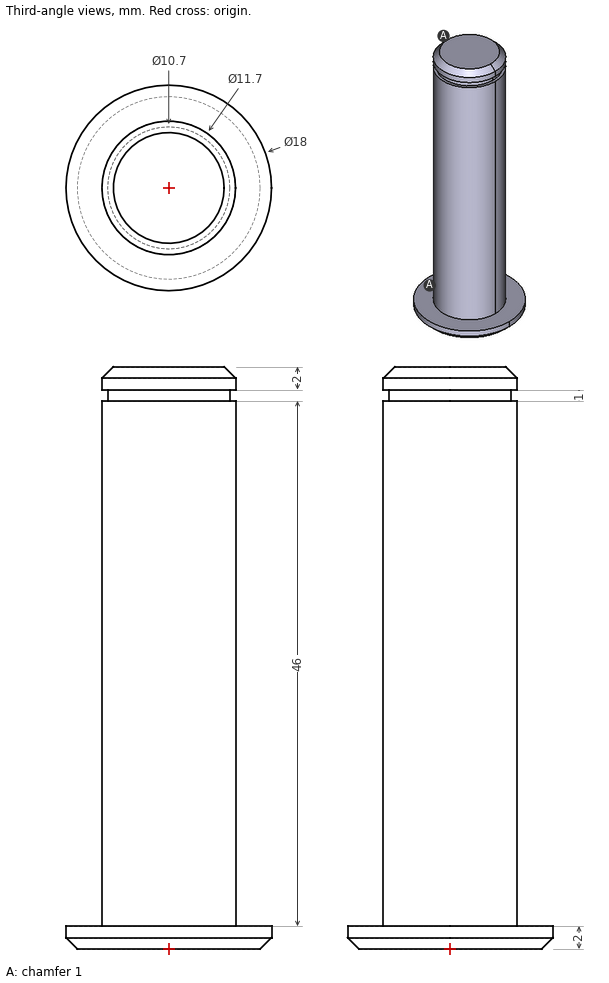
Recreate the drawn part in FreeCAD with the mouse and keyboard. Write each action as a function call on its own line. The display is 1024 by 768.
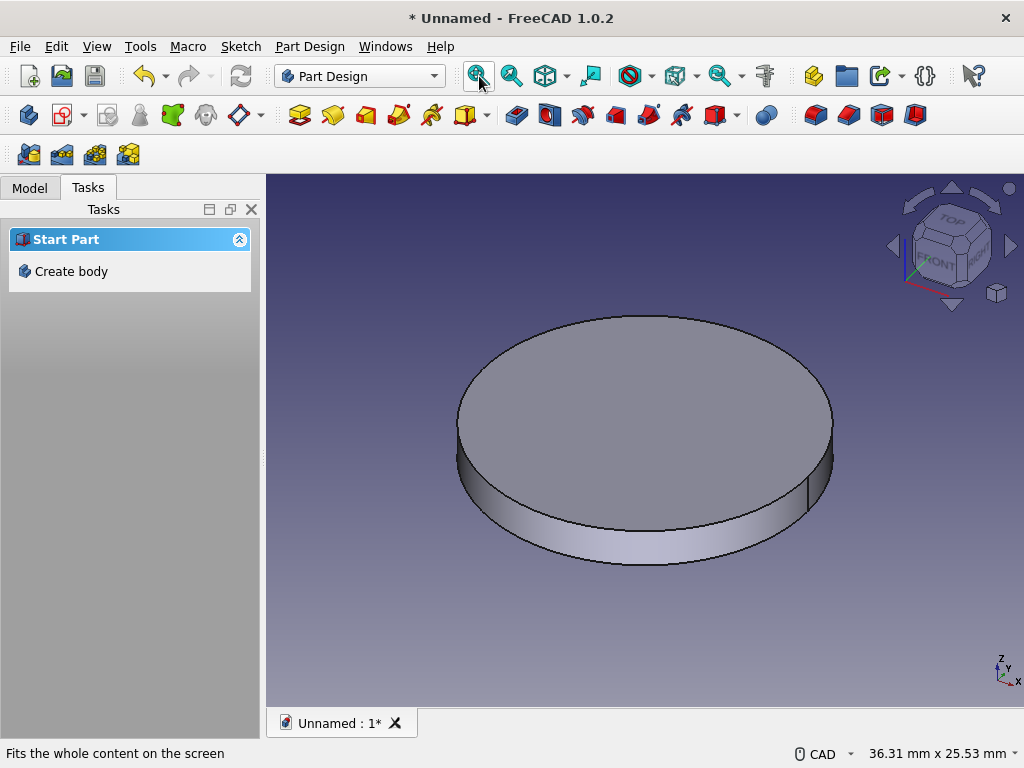
click(645, 422)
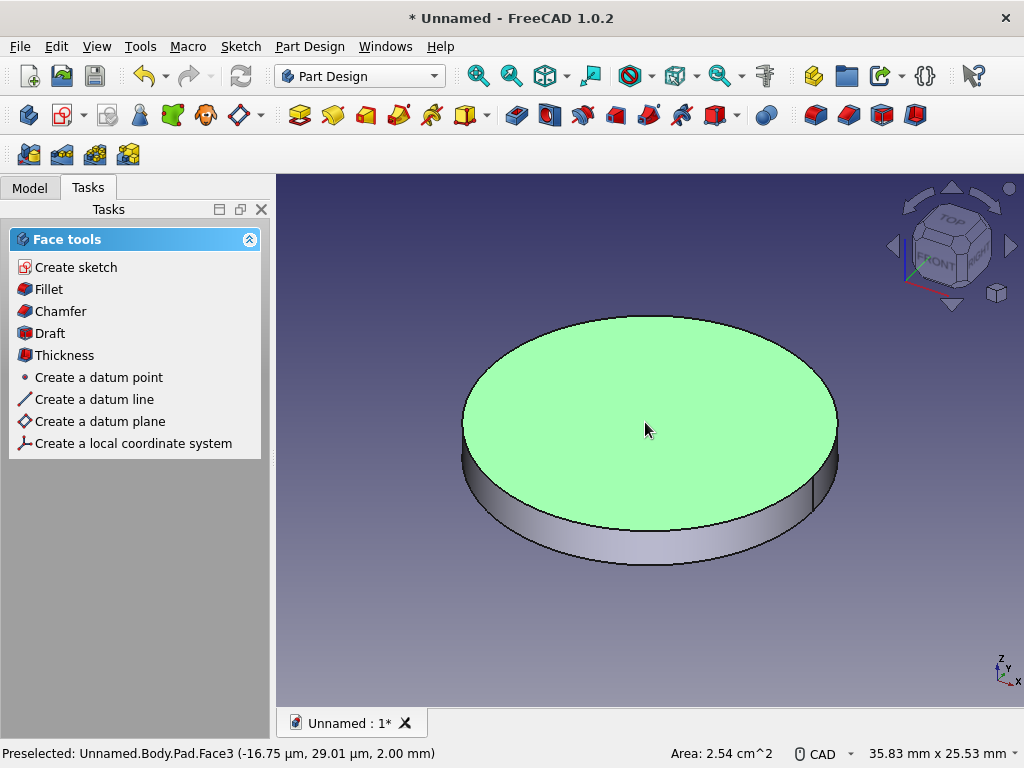
click(62, 116)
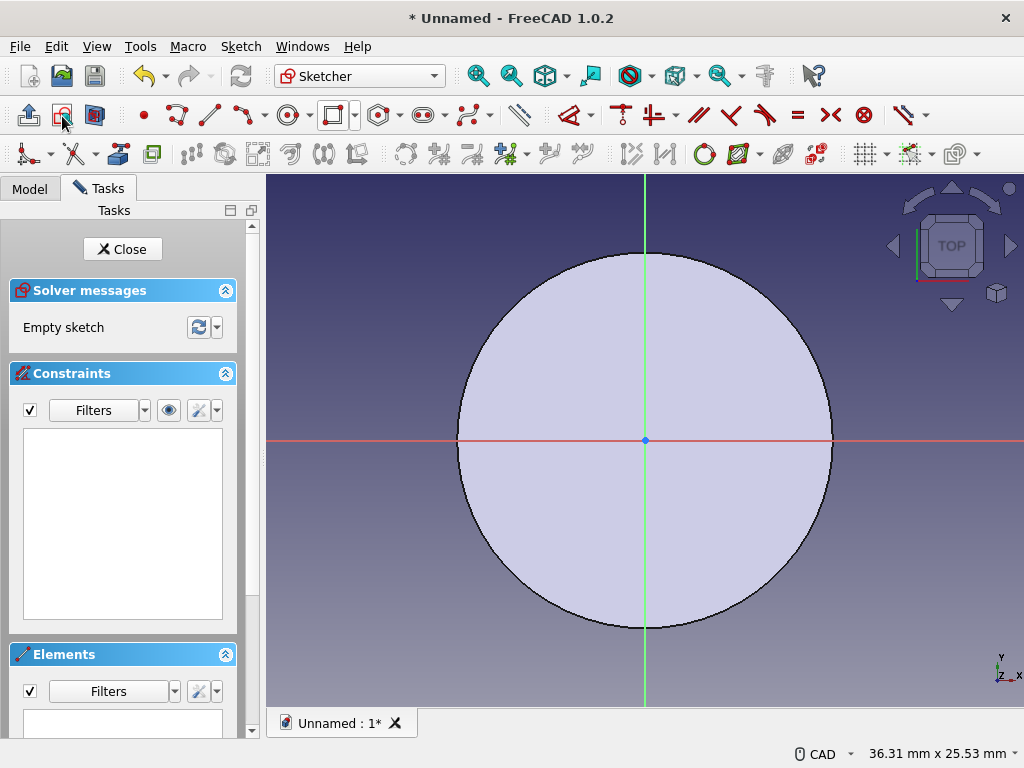
scroll(784, 440, up, 2)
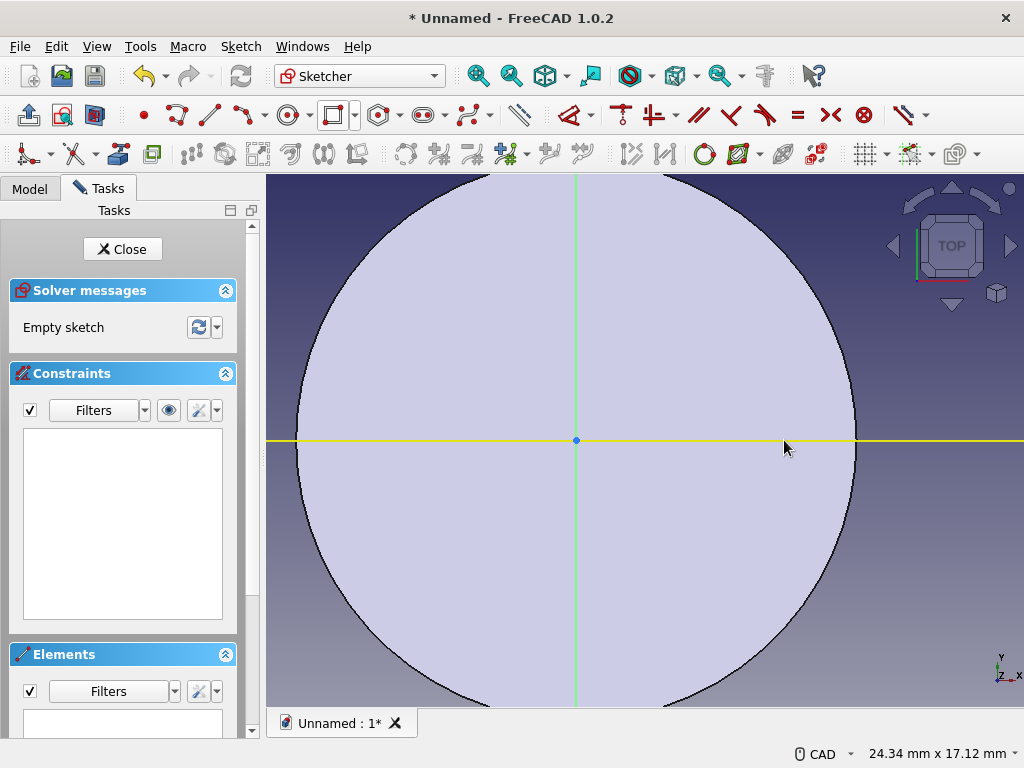
click(288, 116)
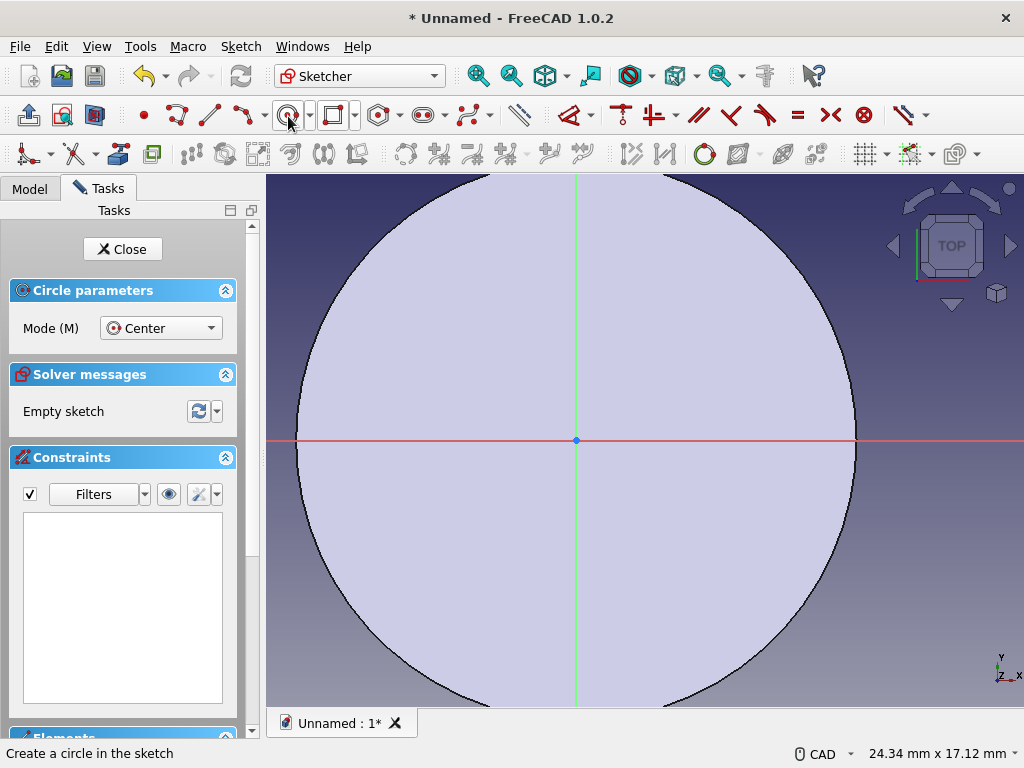
click(576, 440)
move(705, 312)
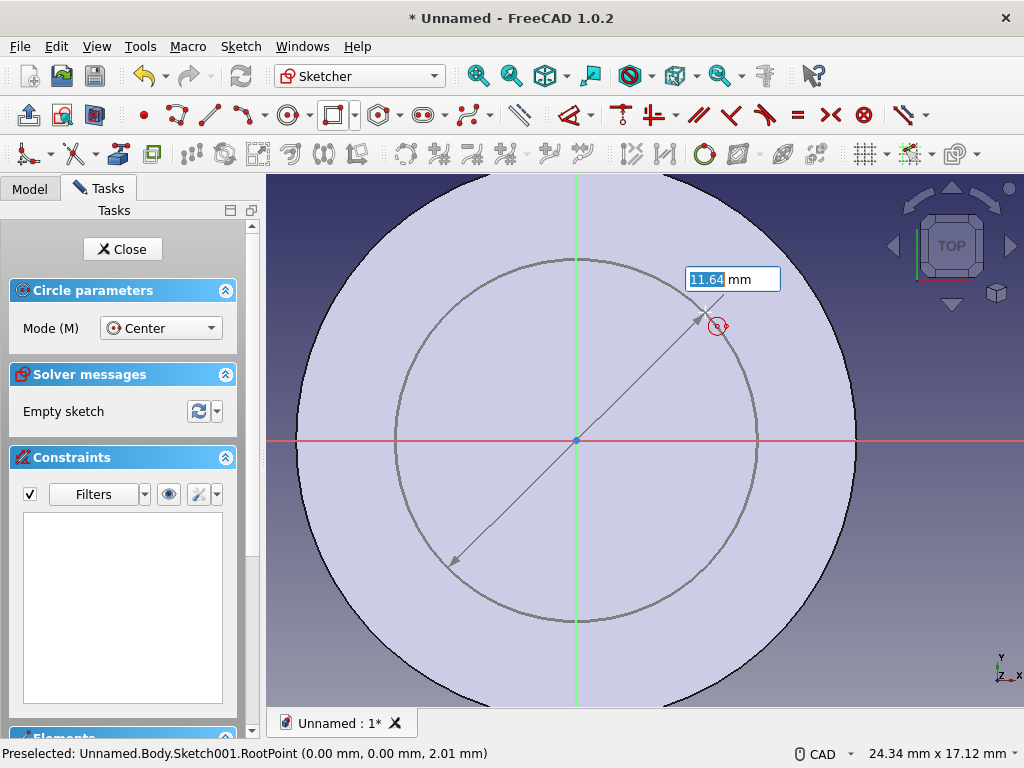
text(11.7)
key(Return)
key(Escape)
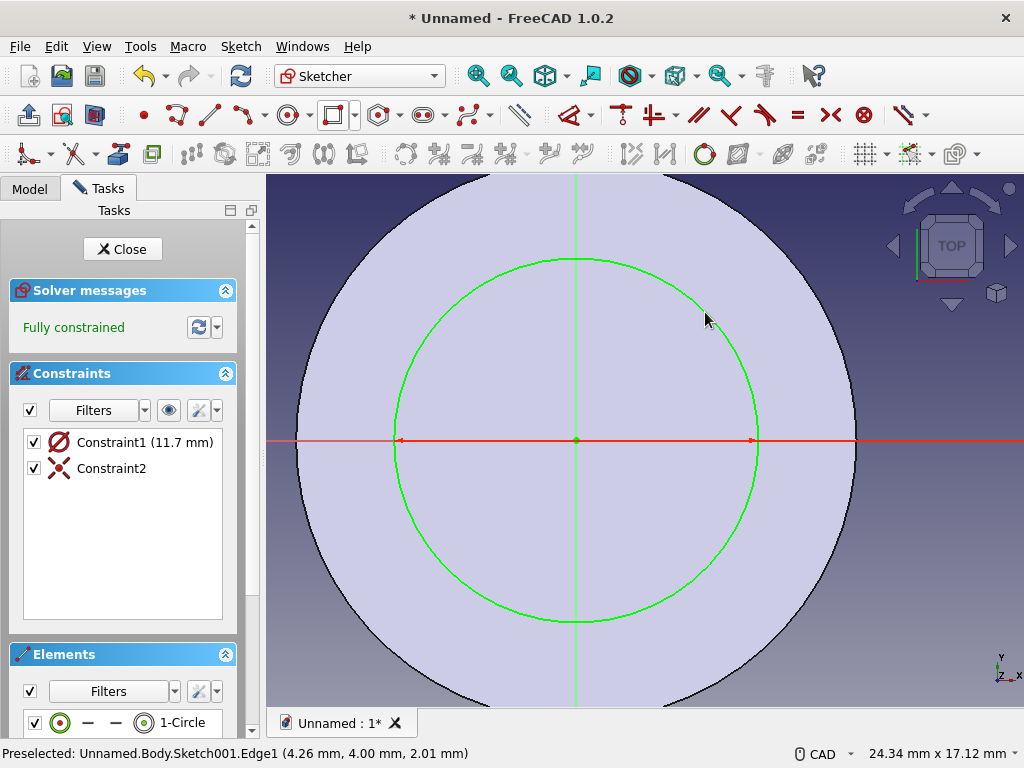
click(123, 249)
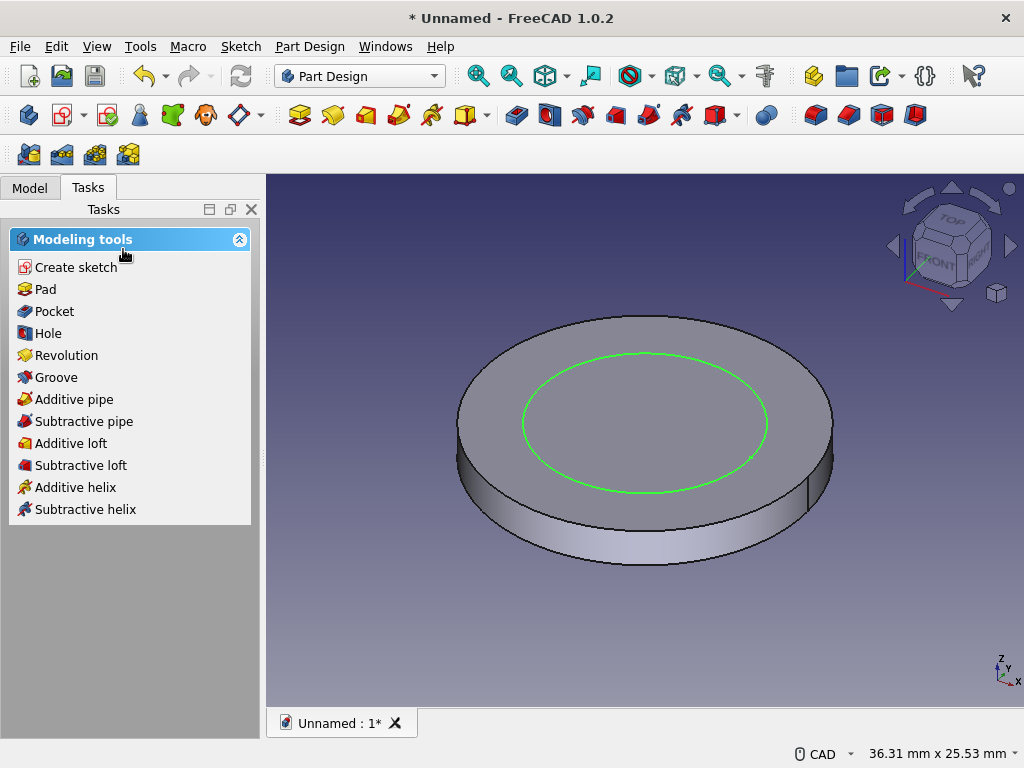
click(300, 116)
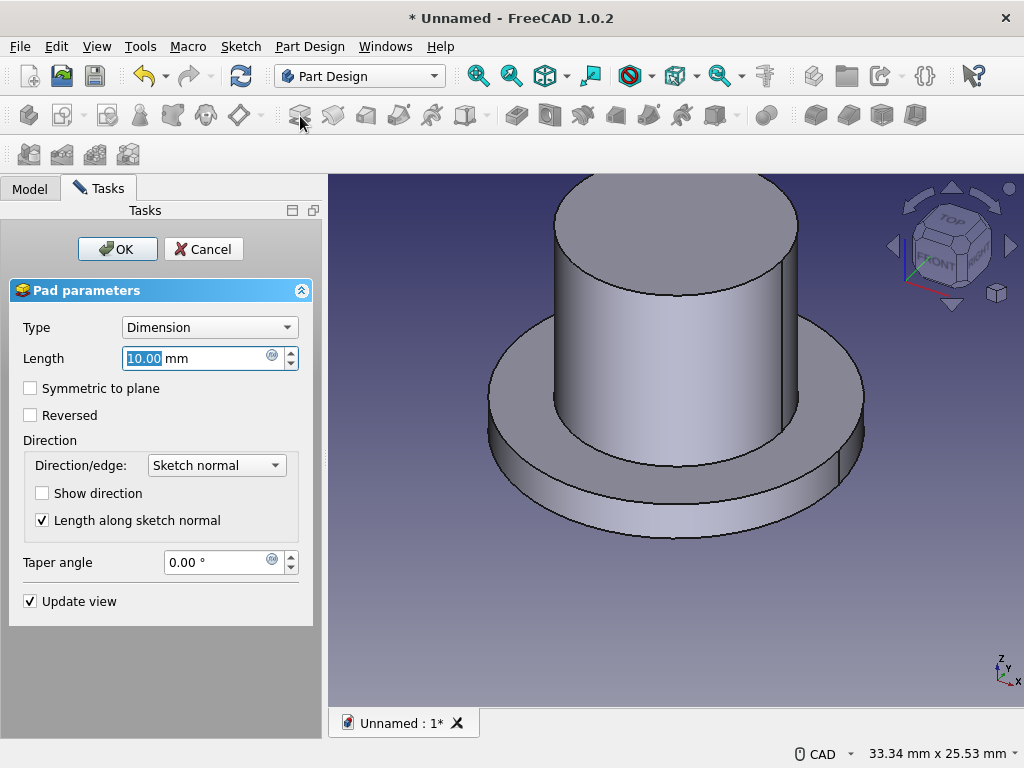
text(46)
key(Tab)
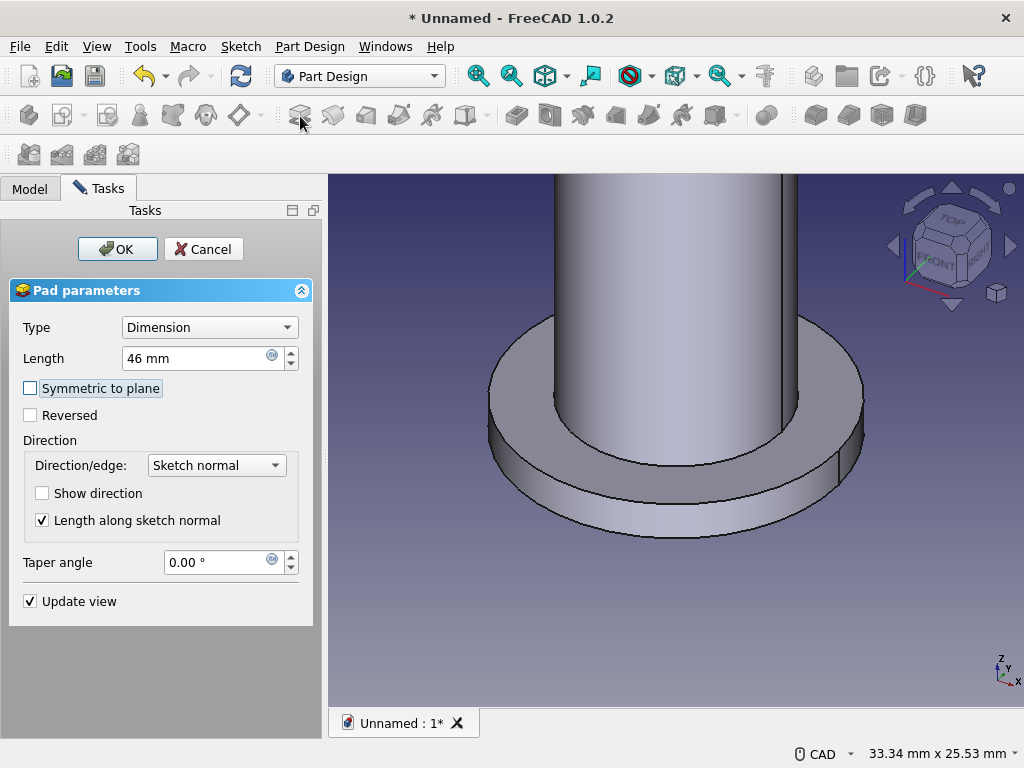
click(118, 249)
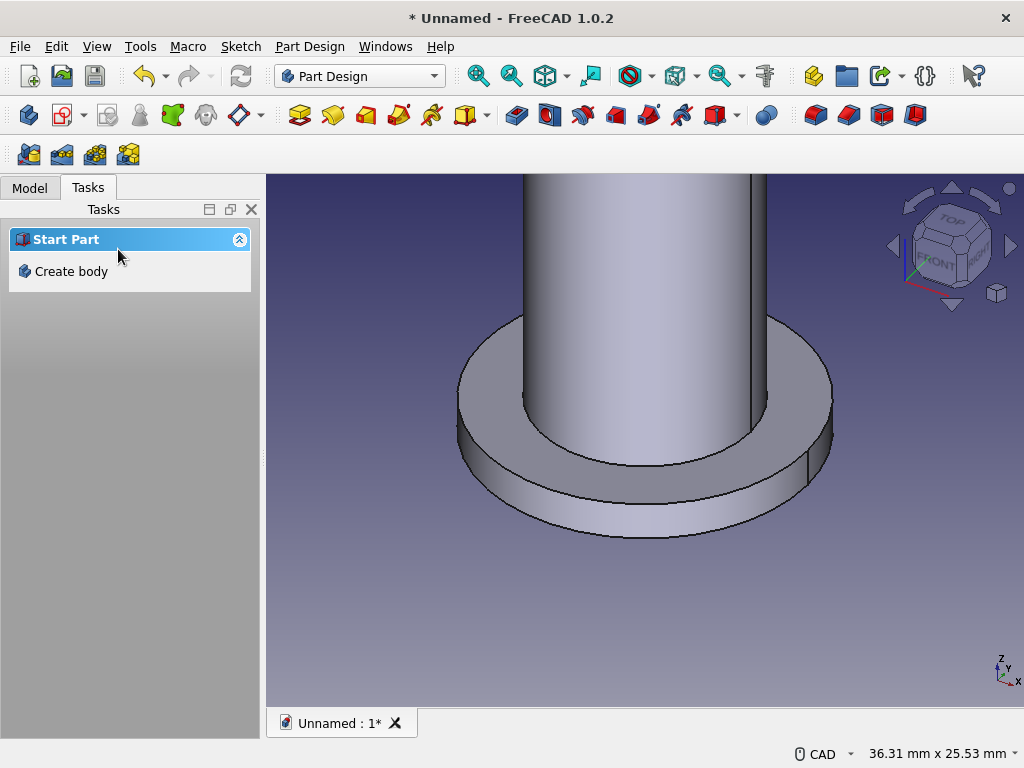
click(479, 76)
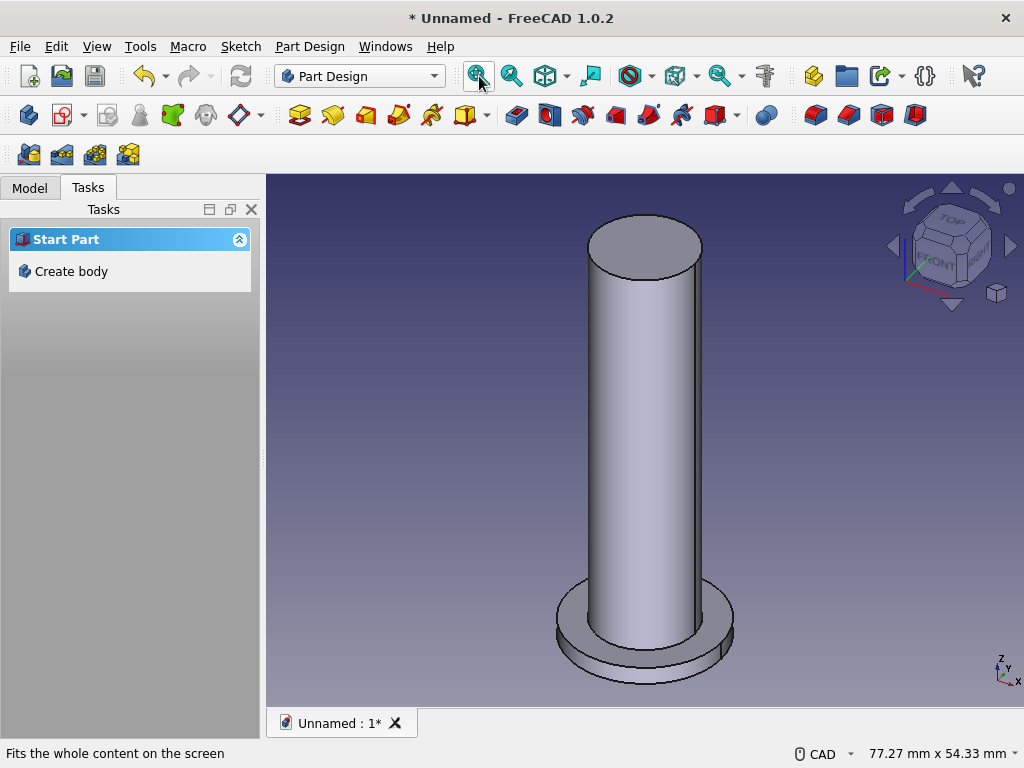
click(645, 247)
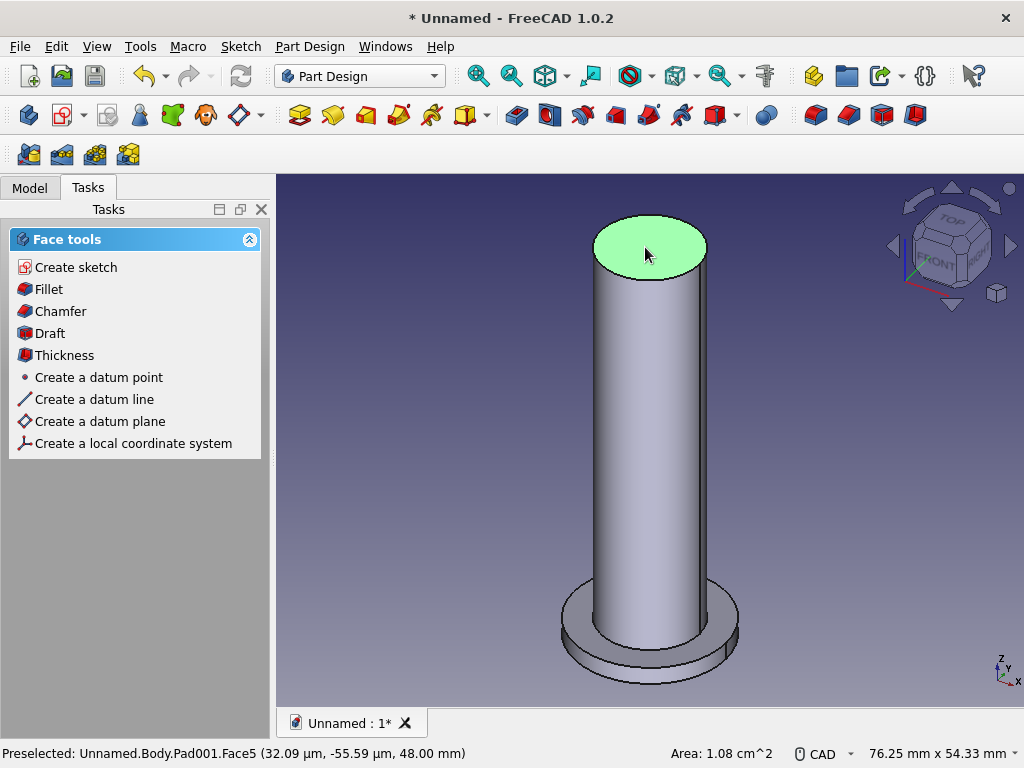
click(62, 116)